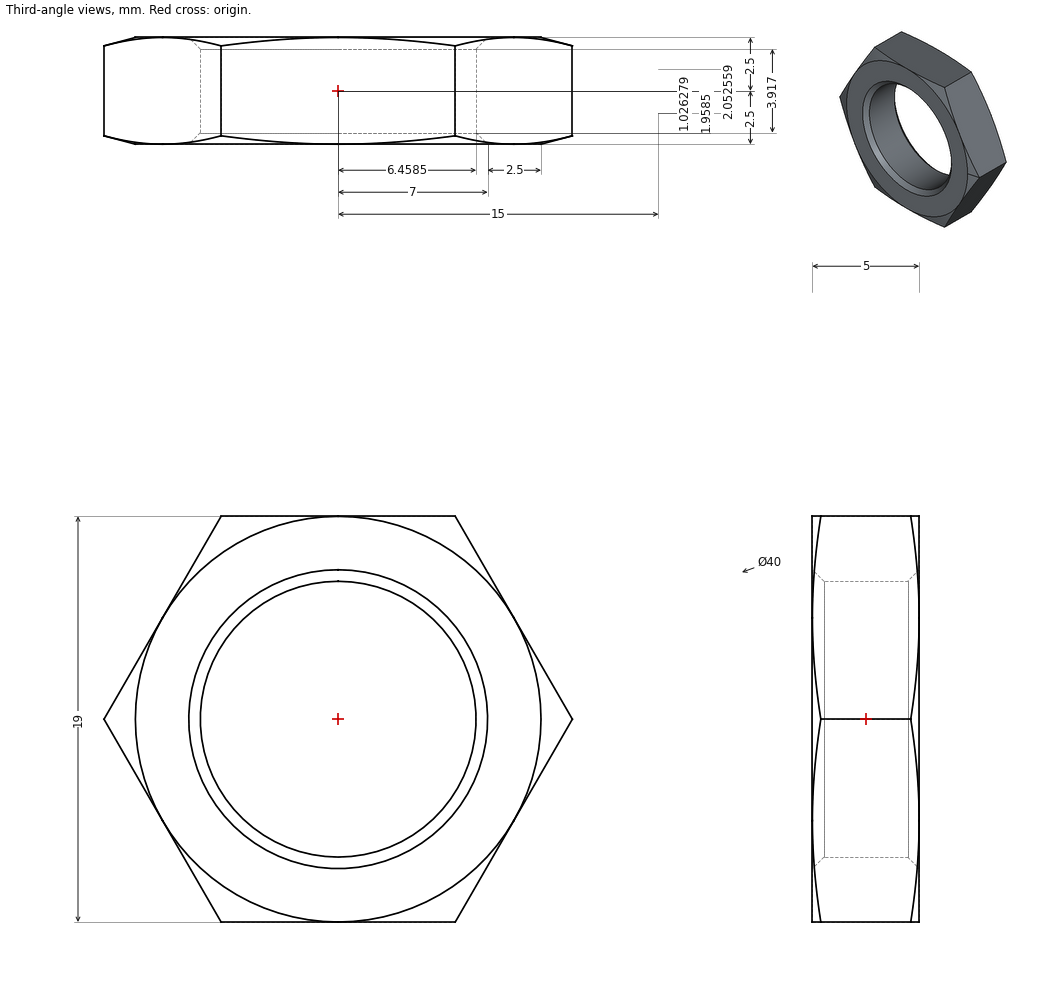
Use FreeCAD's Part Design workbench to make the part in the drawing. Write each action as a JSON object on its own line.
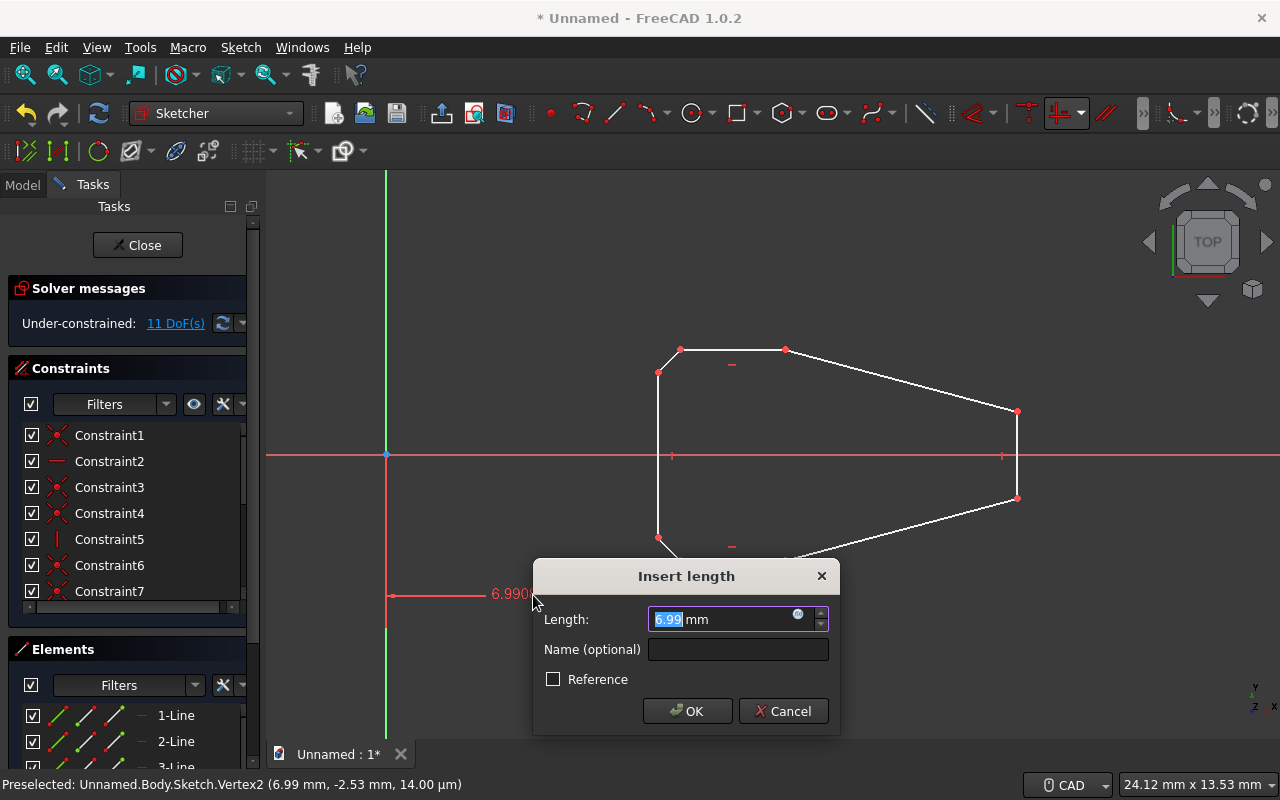
{"action": "type", "text": "7"}
{"action": "key", "text": "Return"}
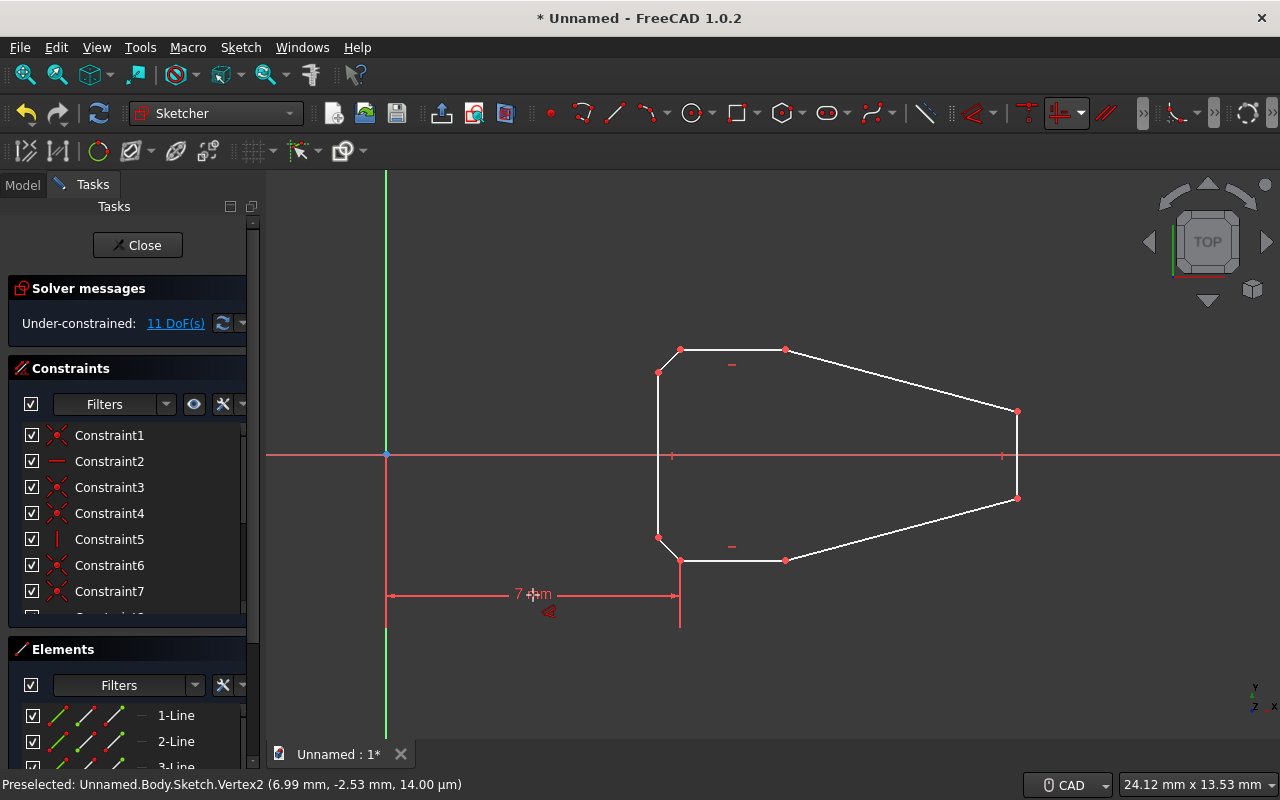
{"action": "left_click", "coordinate": [680, 350]}
{"action": "left_click", "coordinate": [533, 316]}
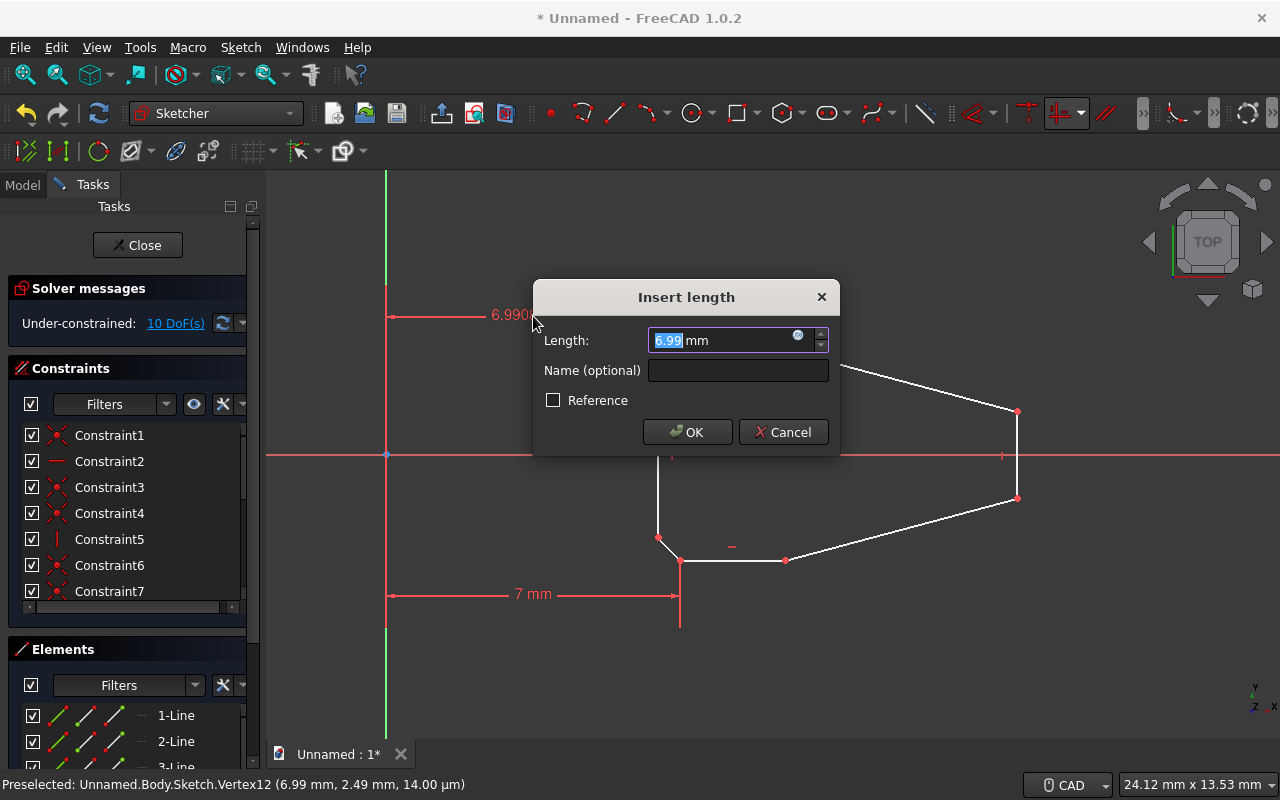
{"action": "type", "text": "7"}
{"action": "key", "text": "Return"}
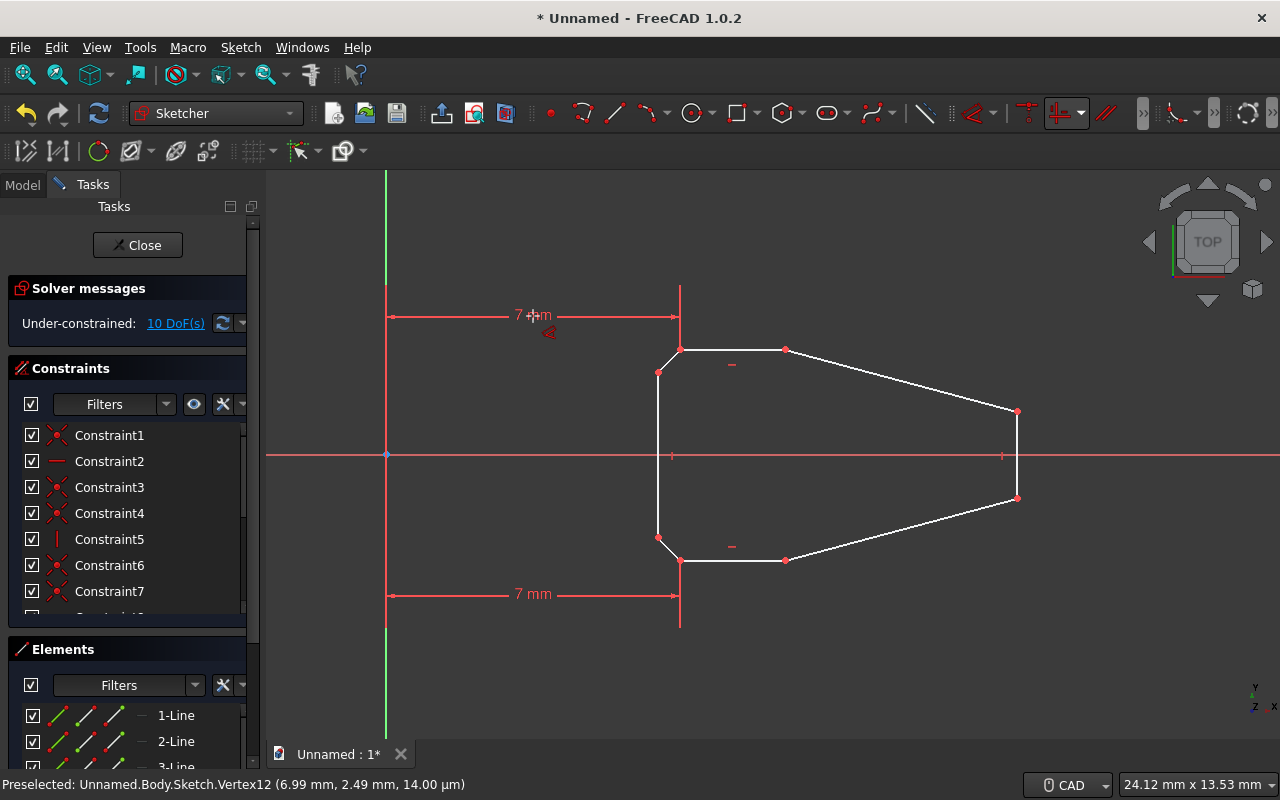
{"action": "left_click", "coordinate": [712, 561]}
{"action": "left_click", "coordinate": [733, 595]}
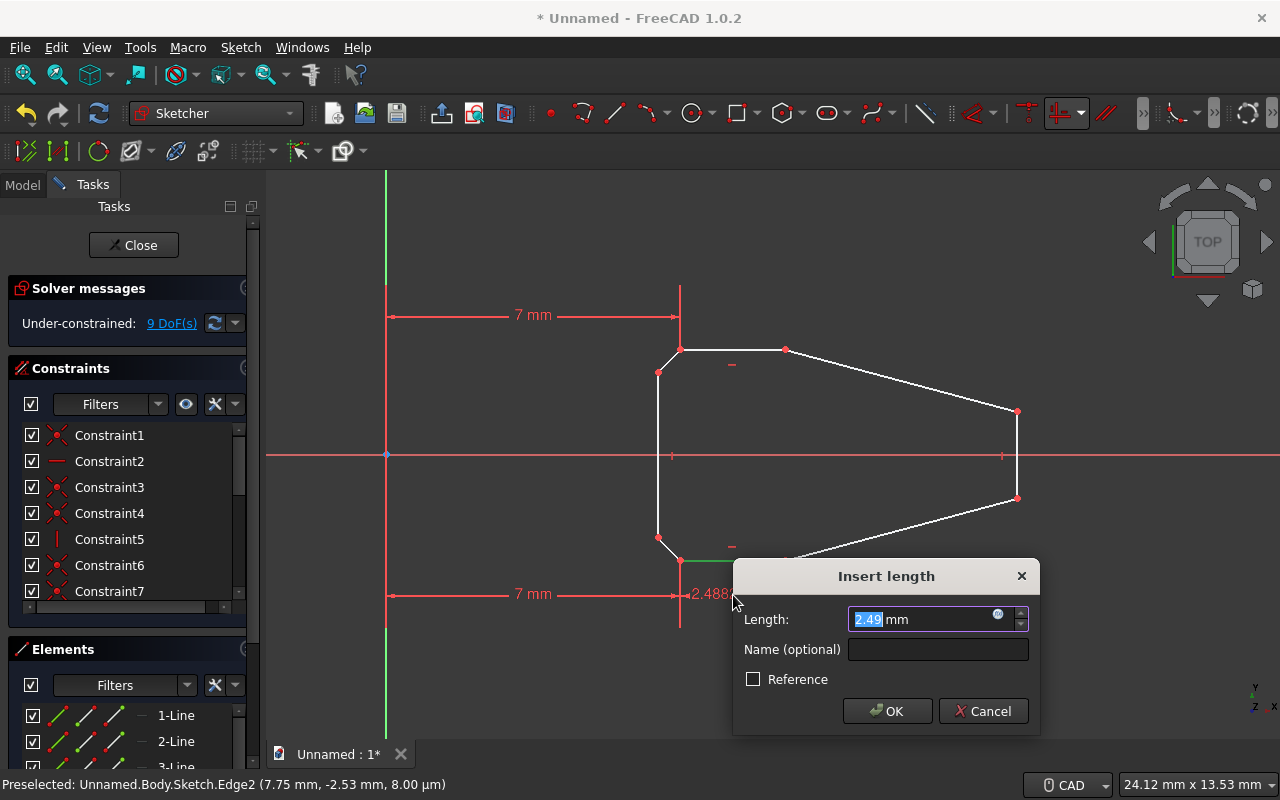
{"action": "type", "text": "2.5"}
{"action": "key", "text": "Return"}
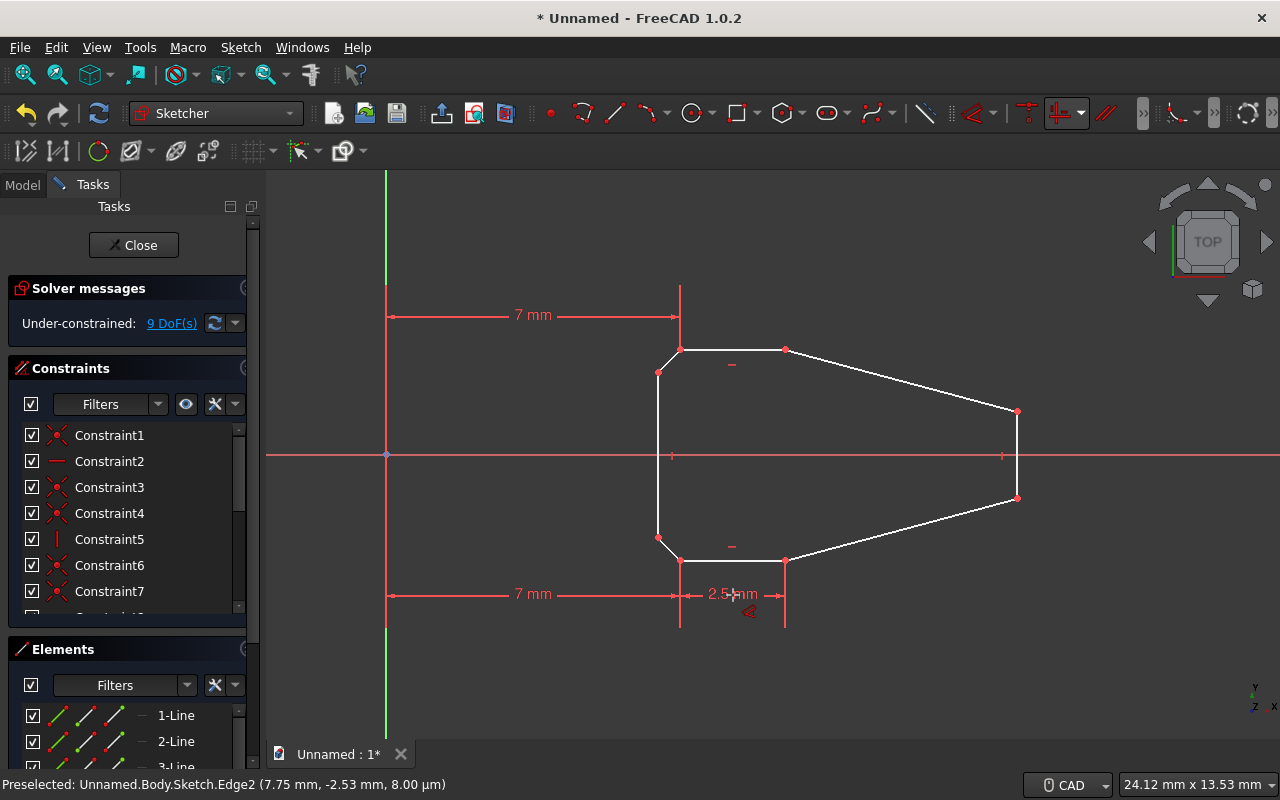
{"action": "left_click", "coordinate": [754, 350]}
{"action": "left_click", "coordinate": [733, 316]}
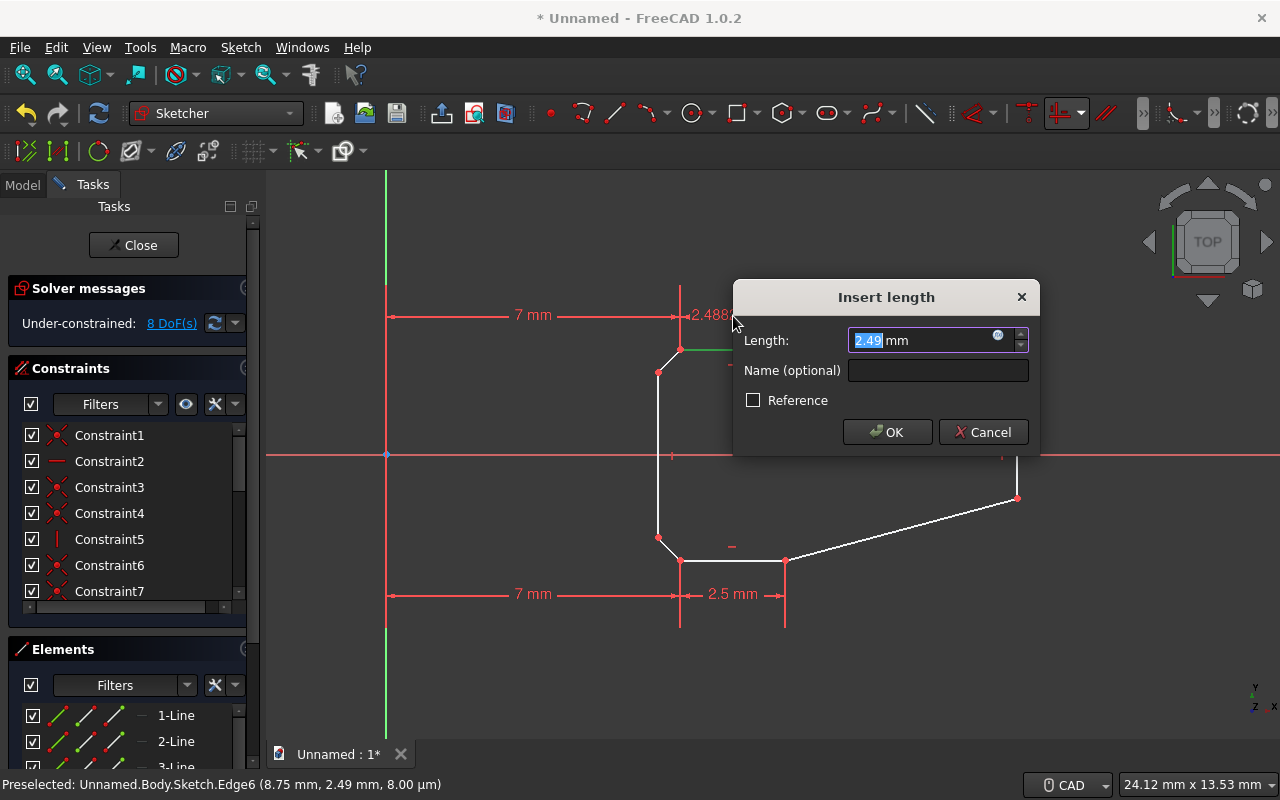
{"action": "type", "text": "2.5"}
{"action": "key", "text": "Return"}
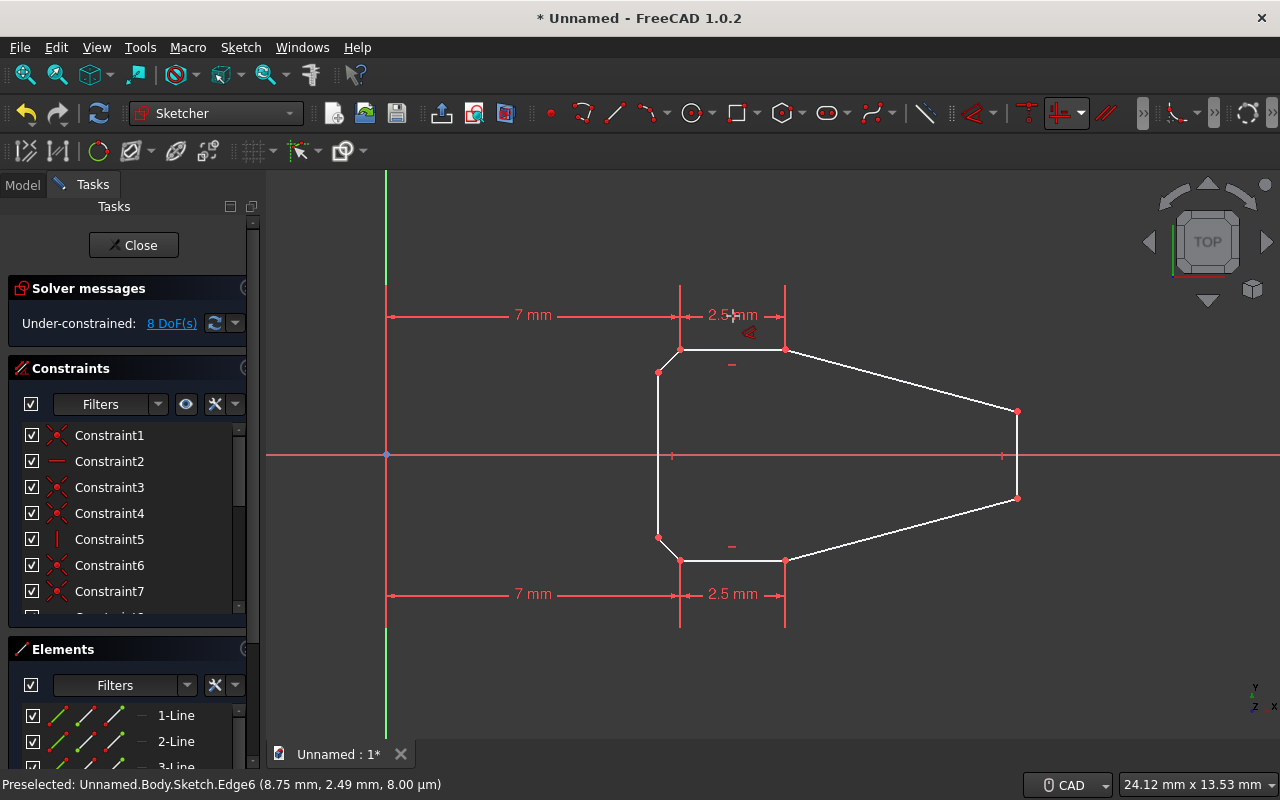
{"action": "left_click", "coordinate": [1017, 499]}
{"action": "left_click", "coordinate": [702, 533]}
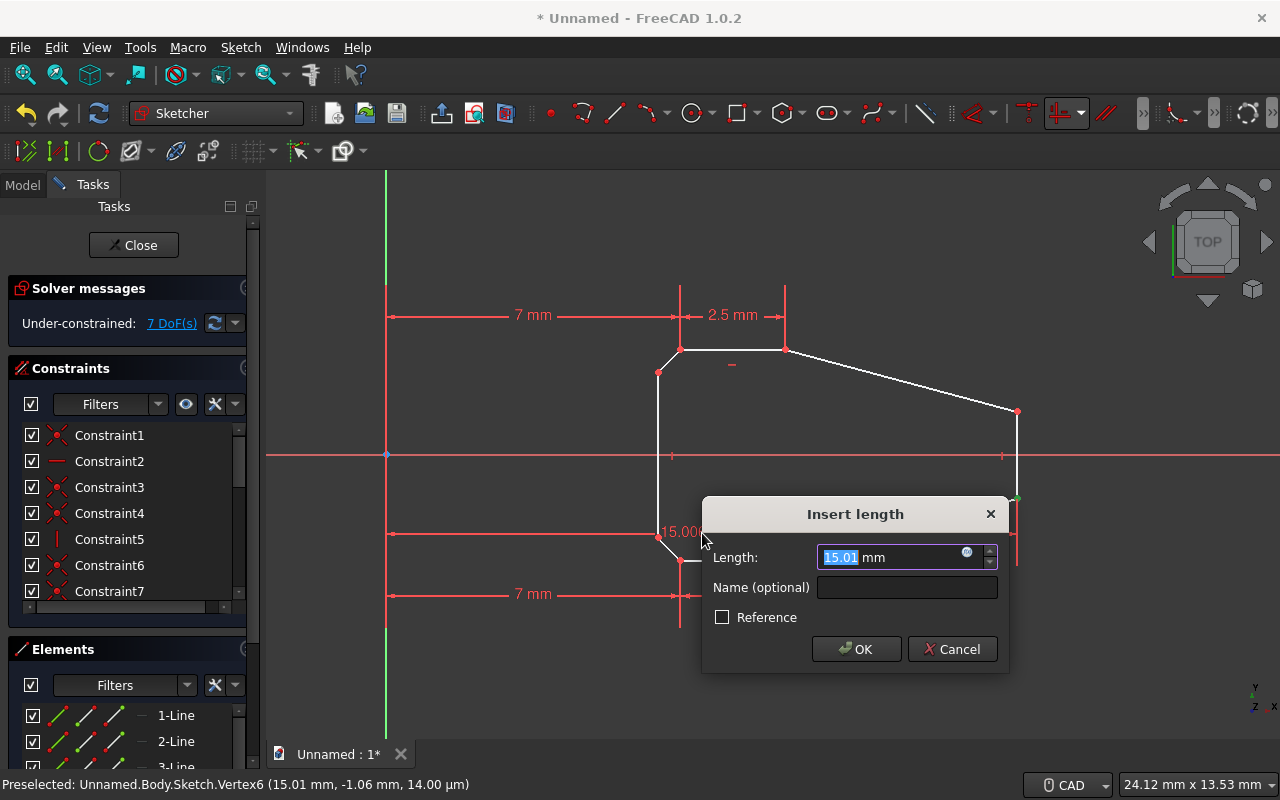
{"action": "type", "text": "15"}
{"action": "key", "text": "Return"}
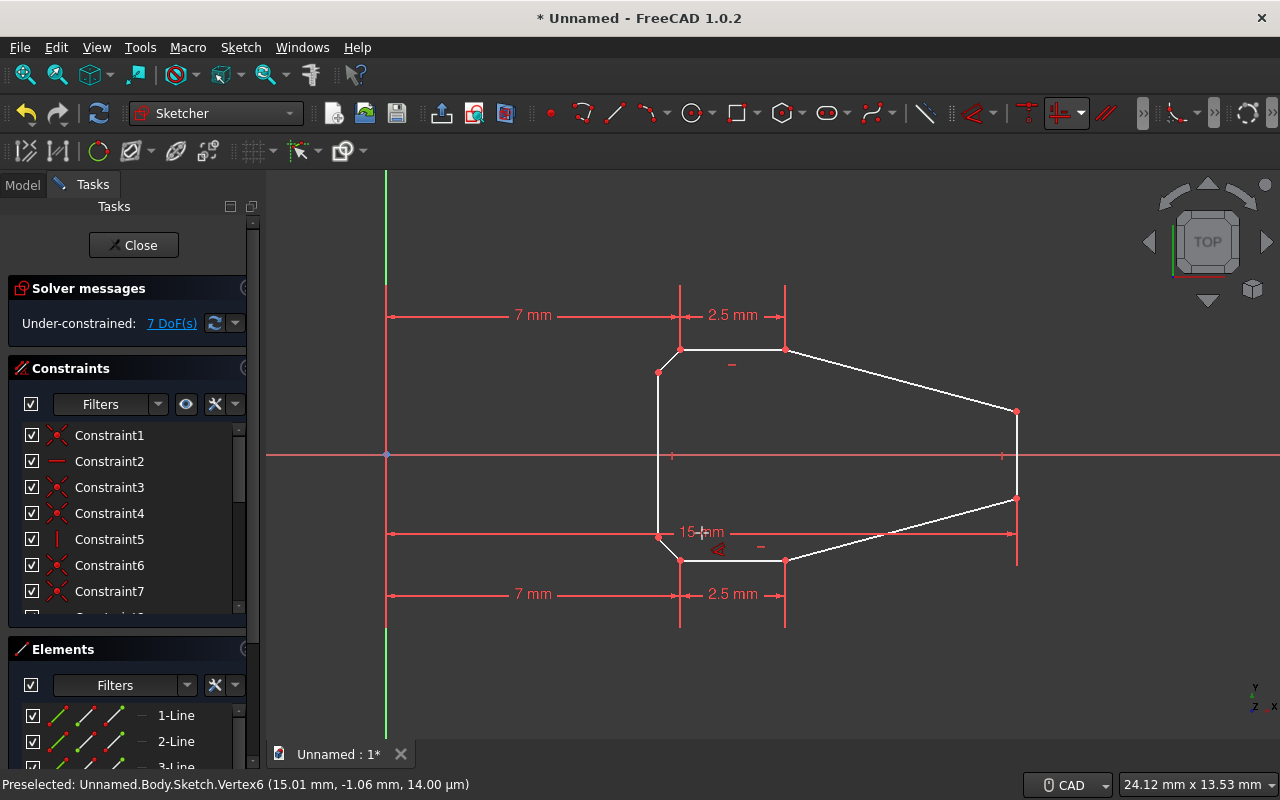
{"action": "left_click", "coordinate": [680, 561]}
{"action": "left_click", "coordinate": [352, 508]}